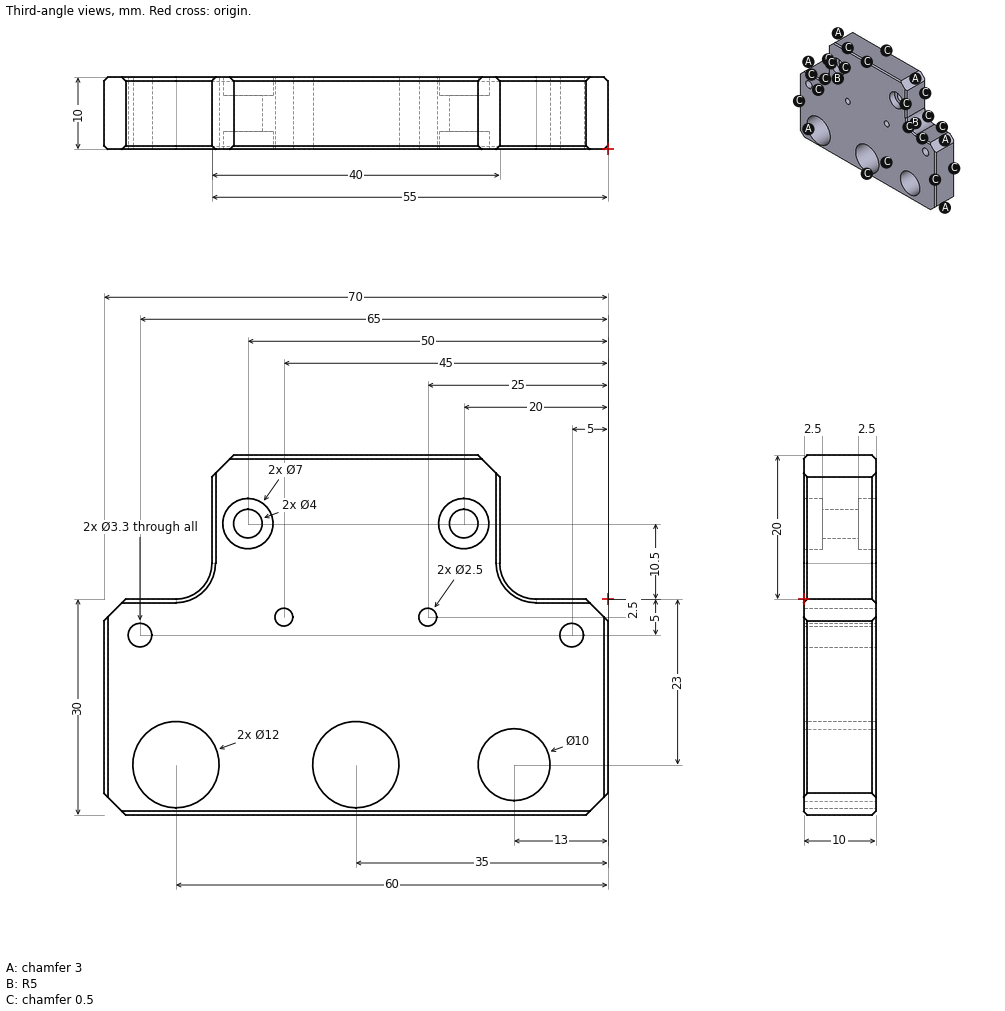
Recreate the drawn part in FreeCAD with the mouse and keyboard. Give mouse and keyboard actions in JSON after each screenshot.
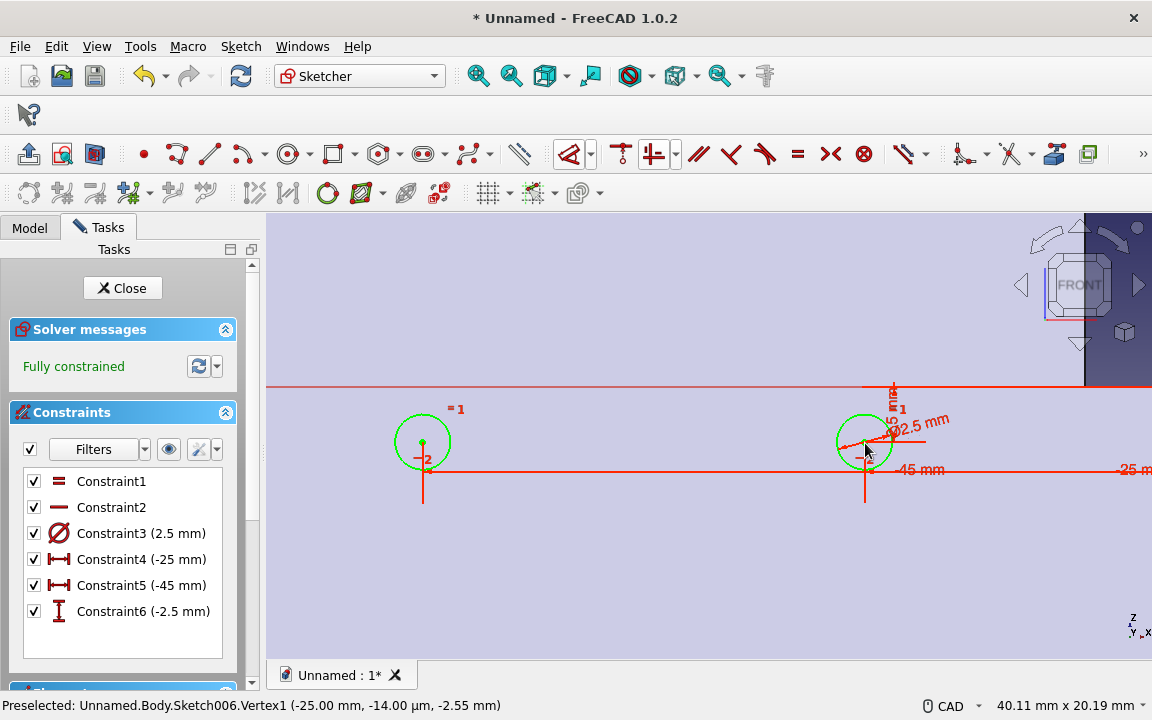
{"action": "left_click", "coordinate": [123, 288]}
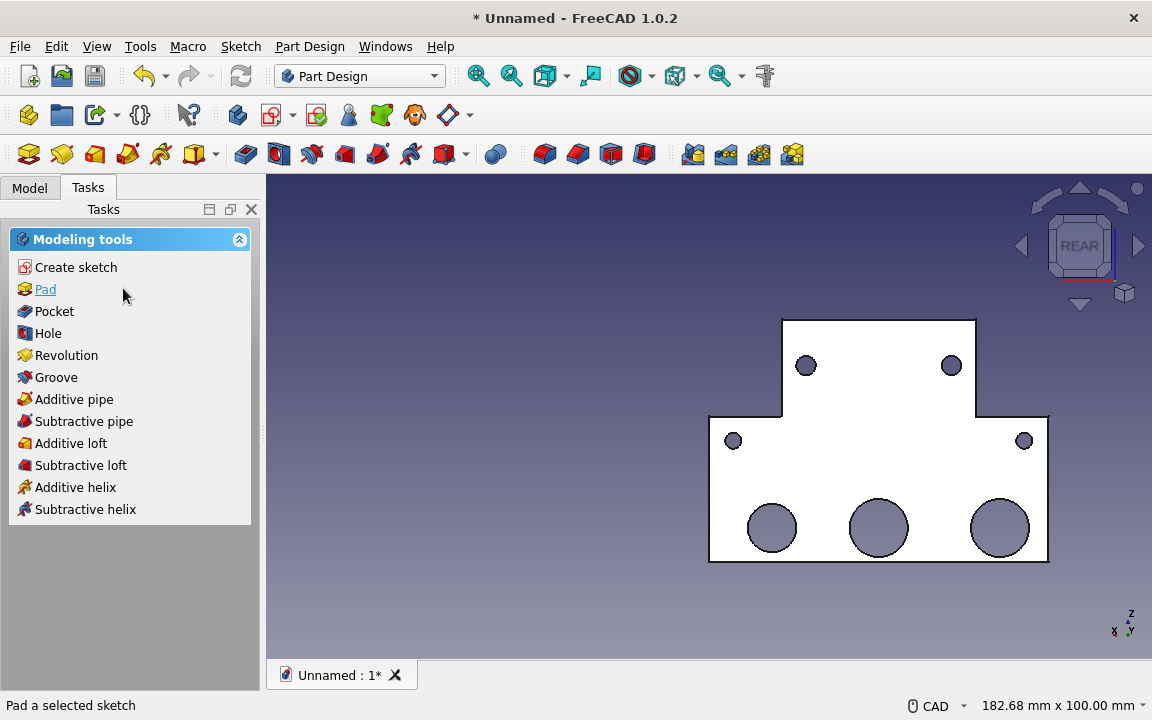
{"action": "left_click", "coordinate": [246, 154]}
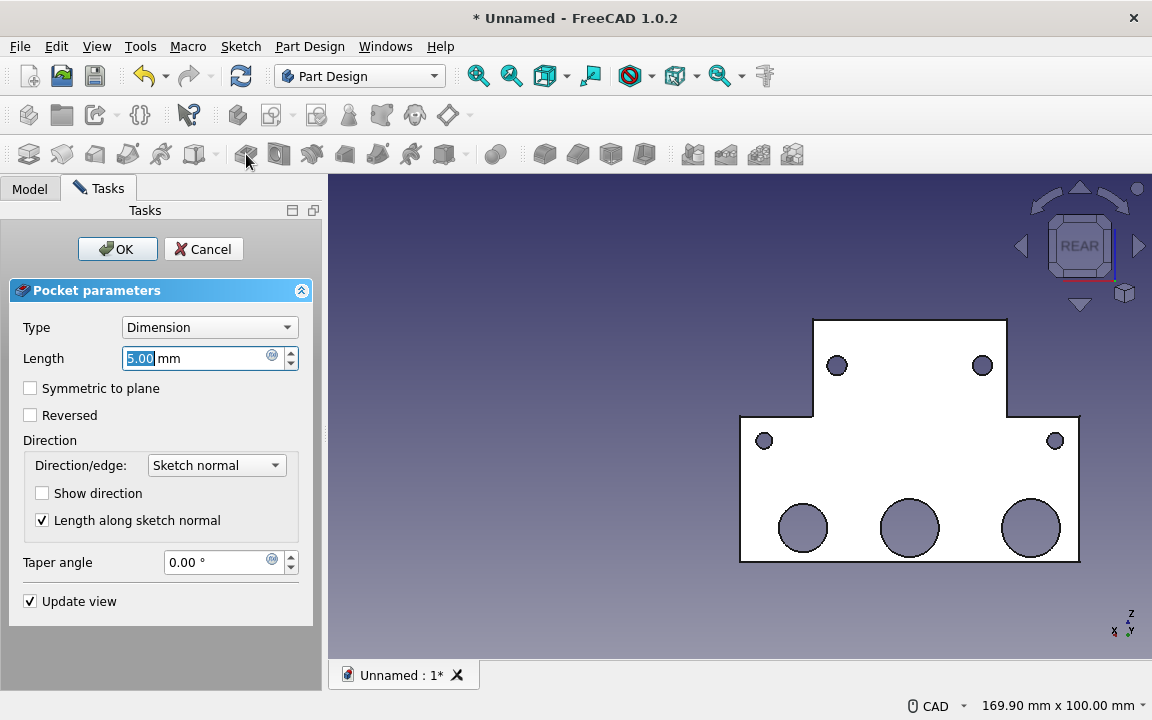
{"action": "left_click", "coordinate": [210, 328]}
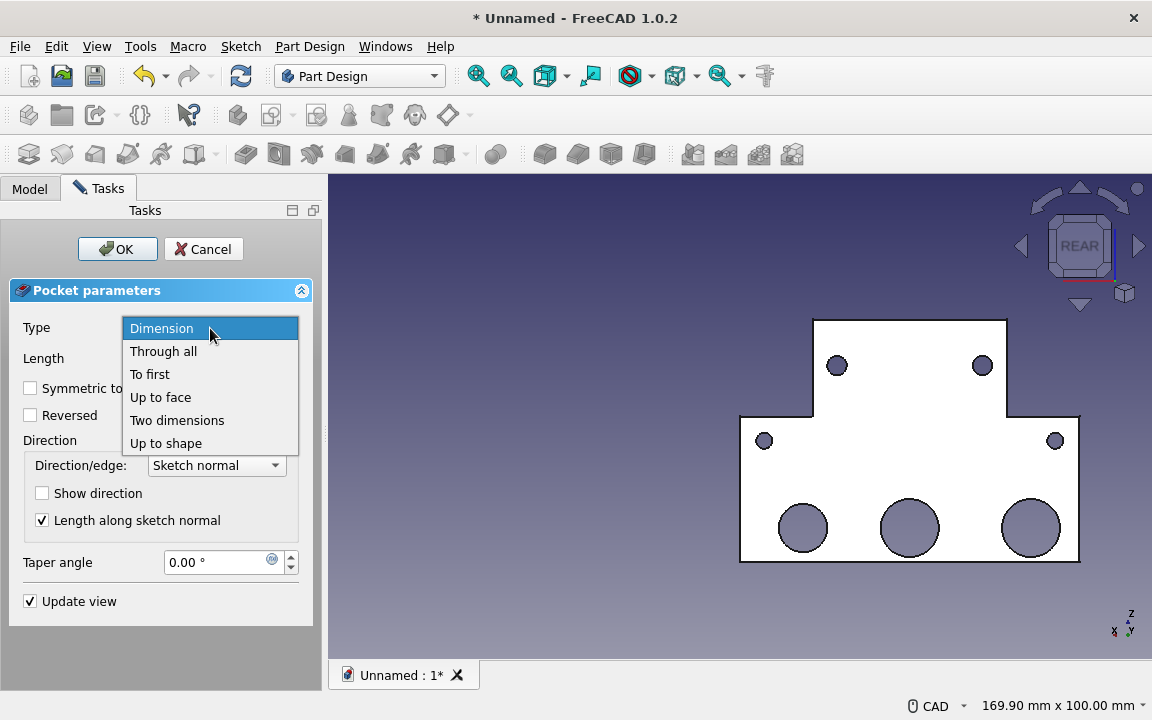
{"action": "left_click", "coordinate": [208, 352]}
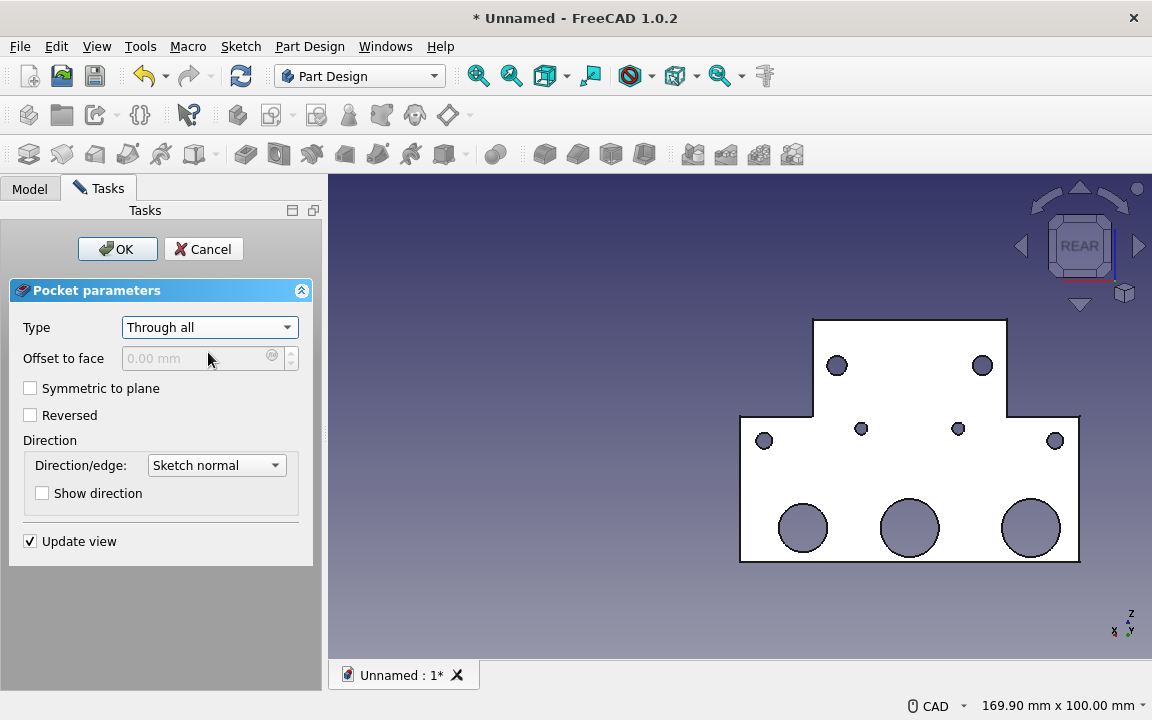
{"action": "left_click", "coordinate": [118, 249]}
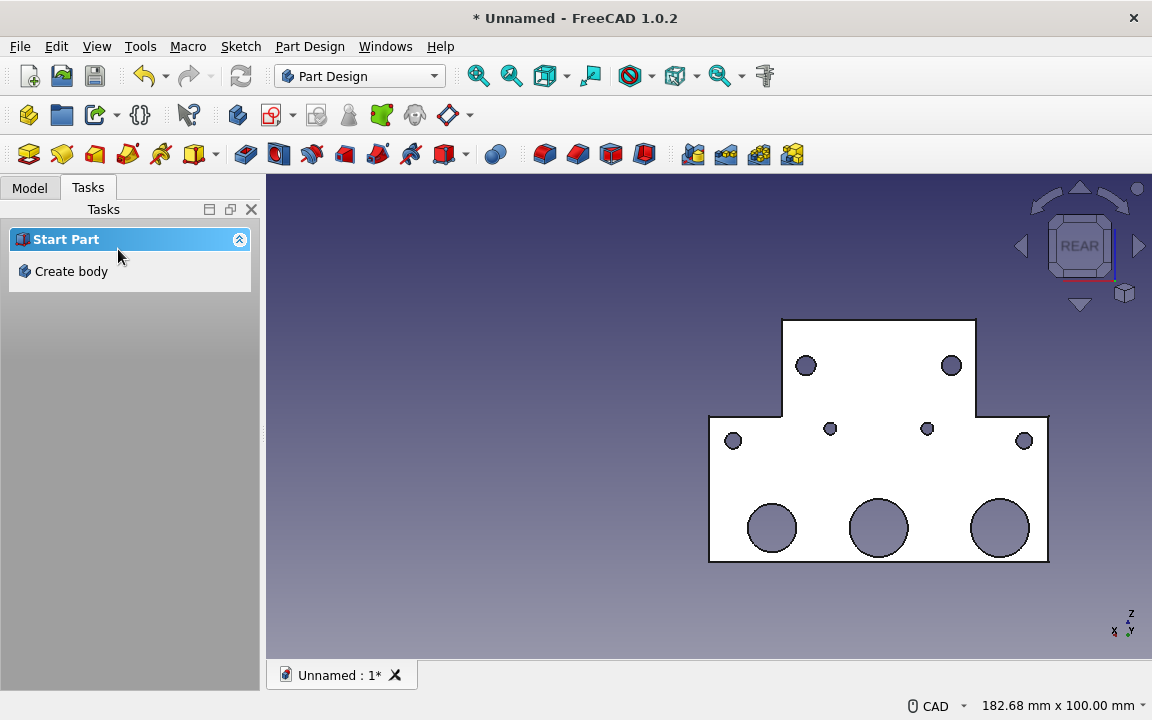
{"action": "key", "text": "0"}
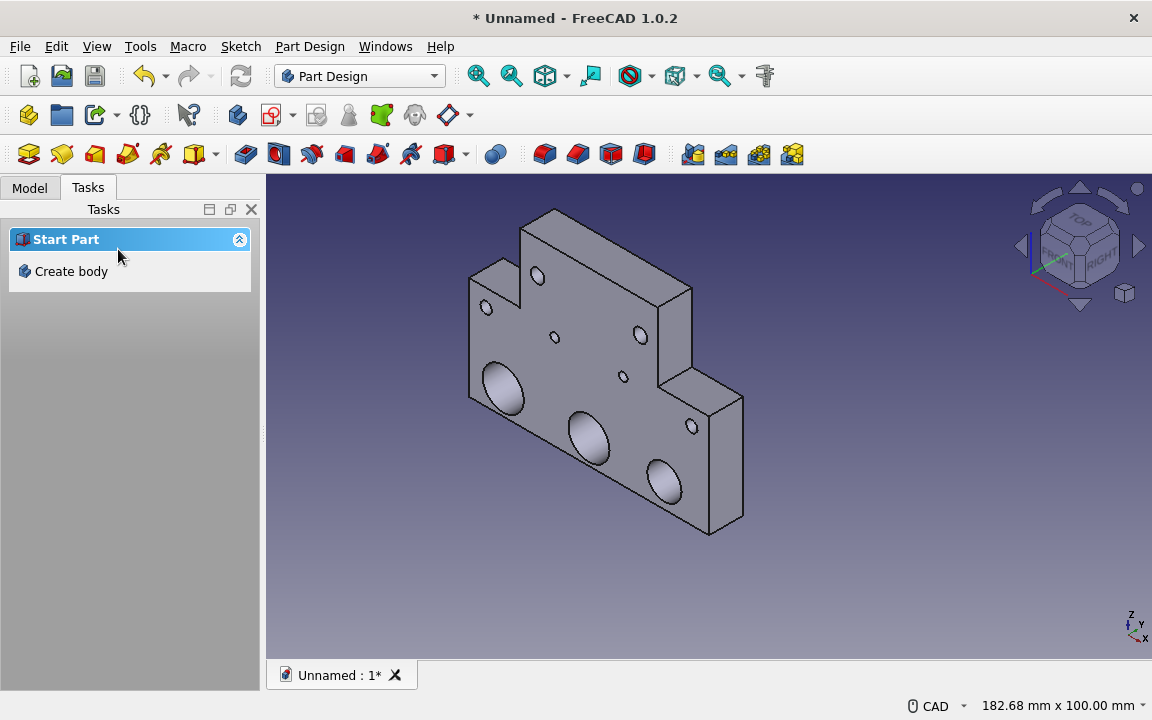
{"action": "left_click", "coordinate": [726, 406]}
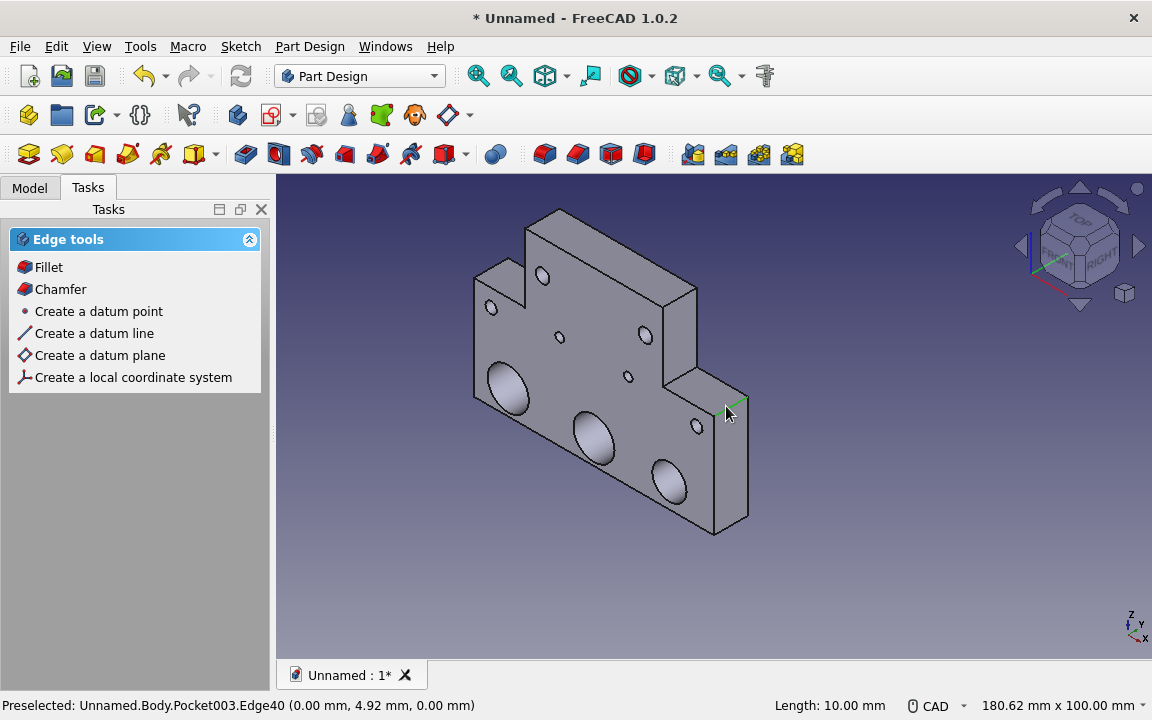
{"action": "left_click", "coordinate": [680, 297], "text": "ctrl"}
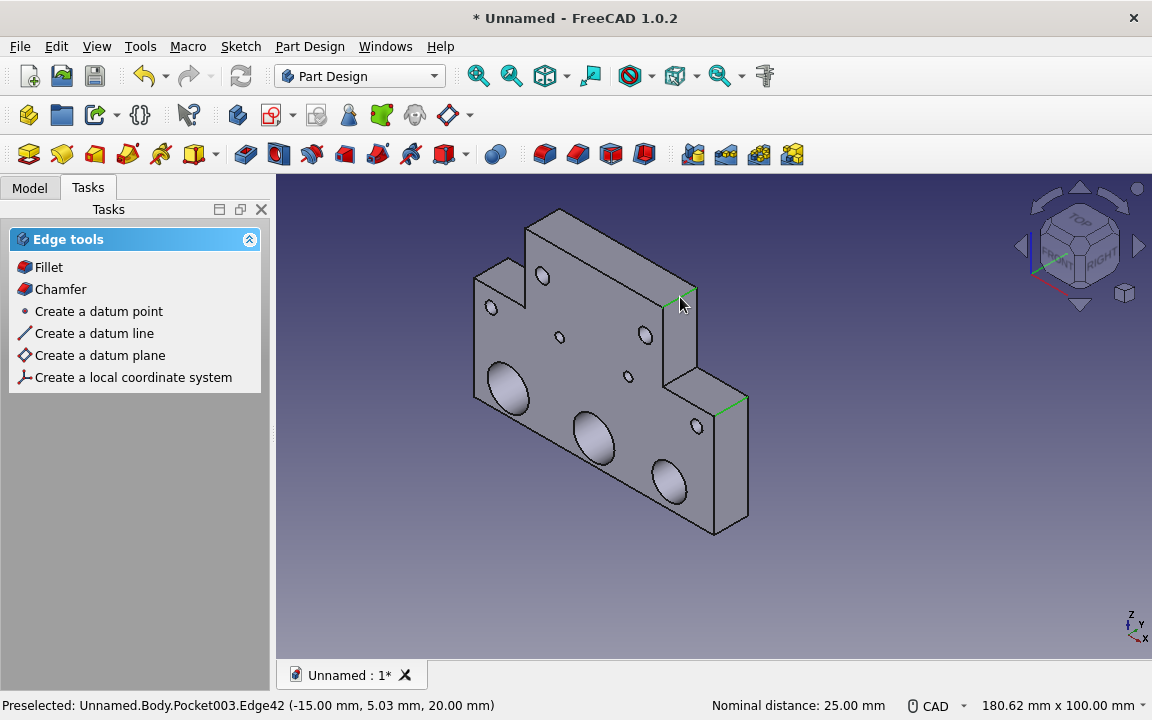
{"action": "key", "text": "2"}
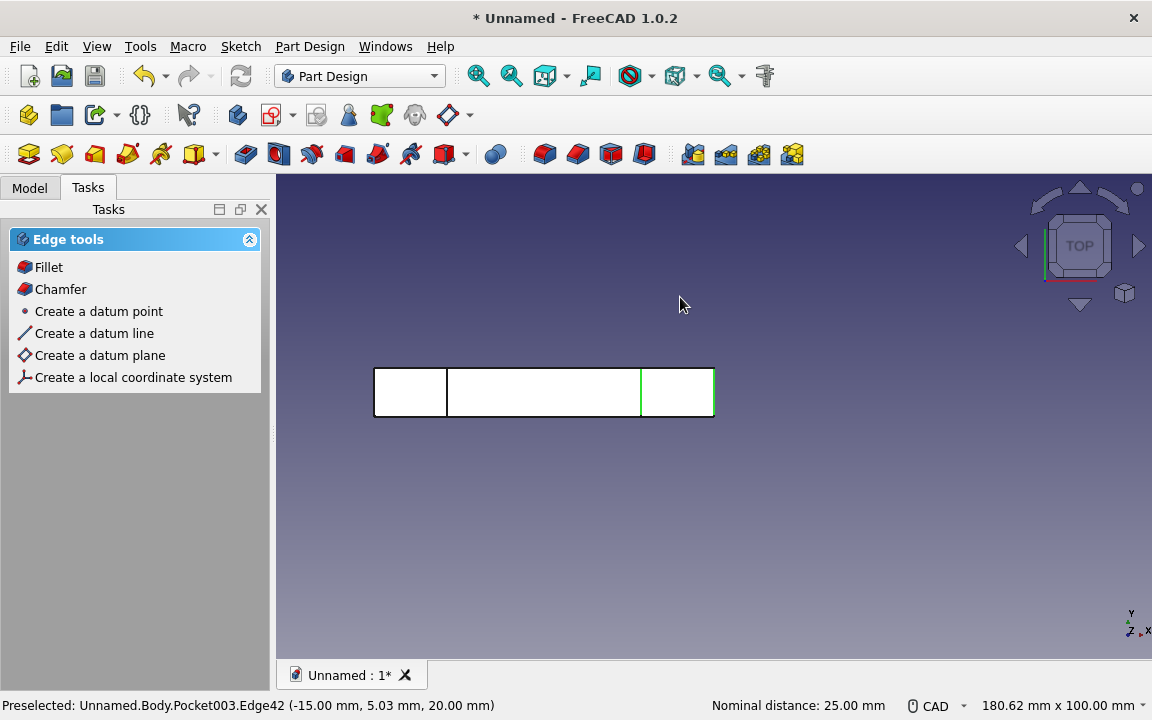
{"action": "left_click", "coordinate": [479, 76]}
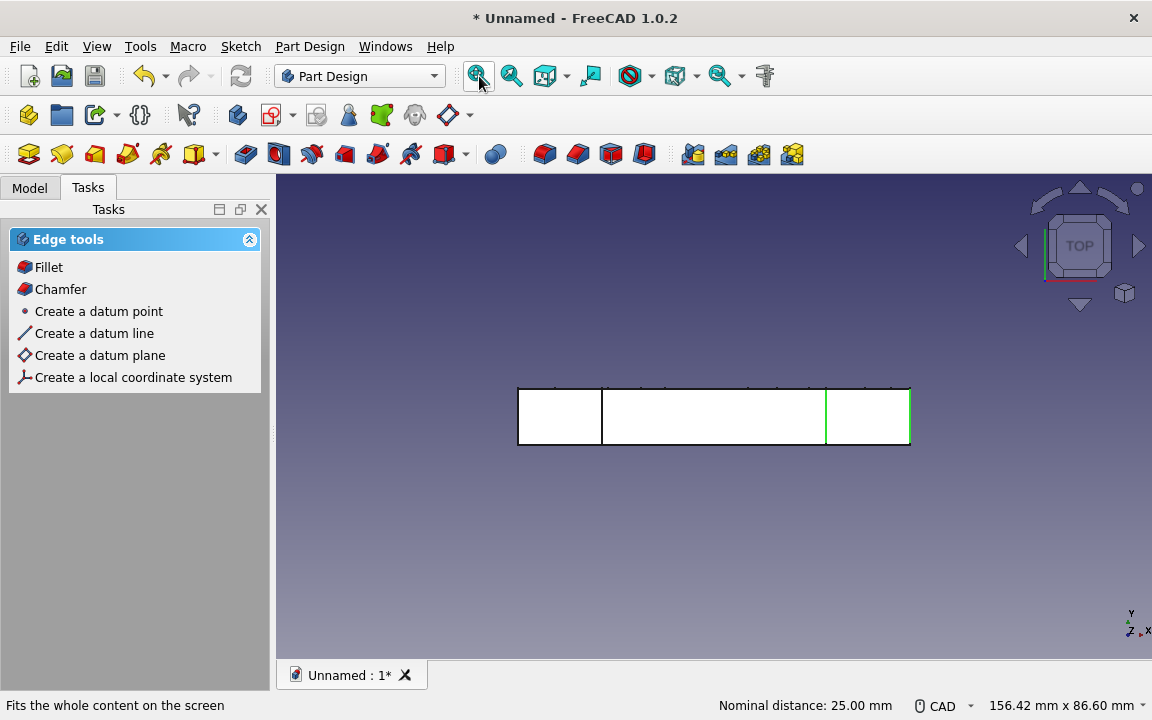
{"action": "left_click", "coordinate": [602, 415], "text": "ctrl"}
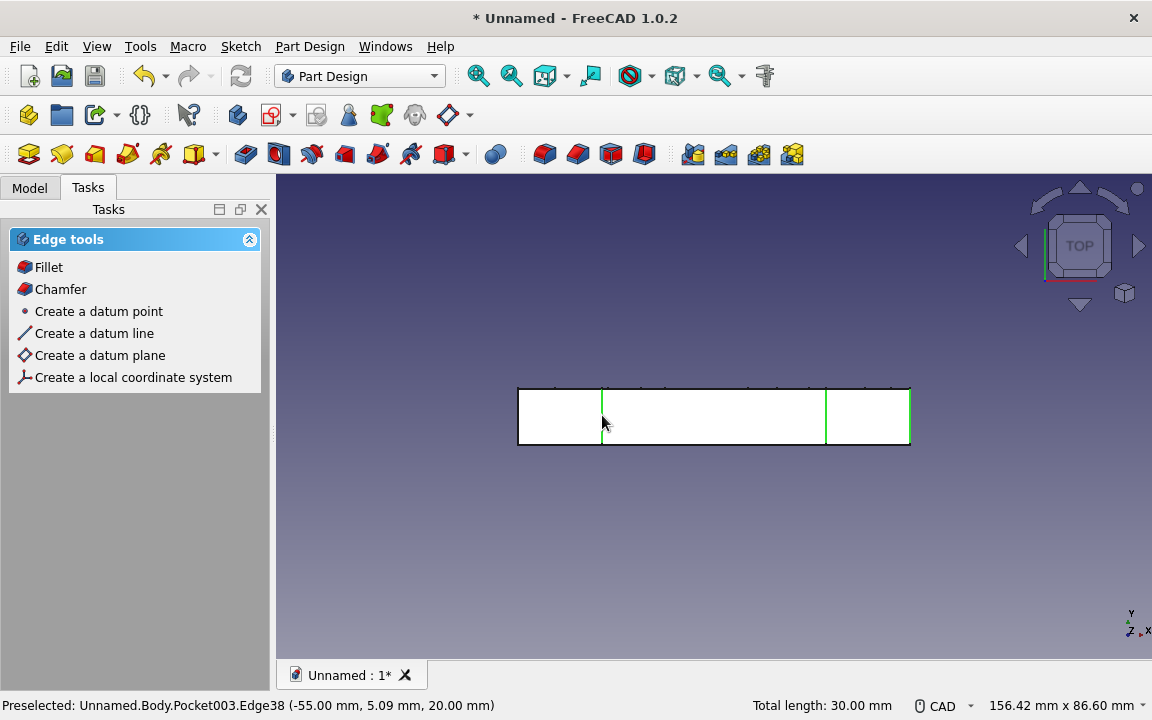
{"action": "left_click", "coordinate": [518, 415], "text": "ctrl"}